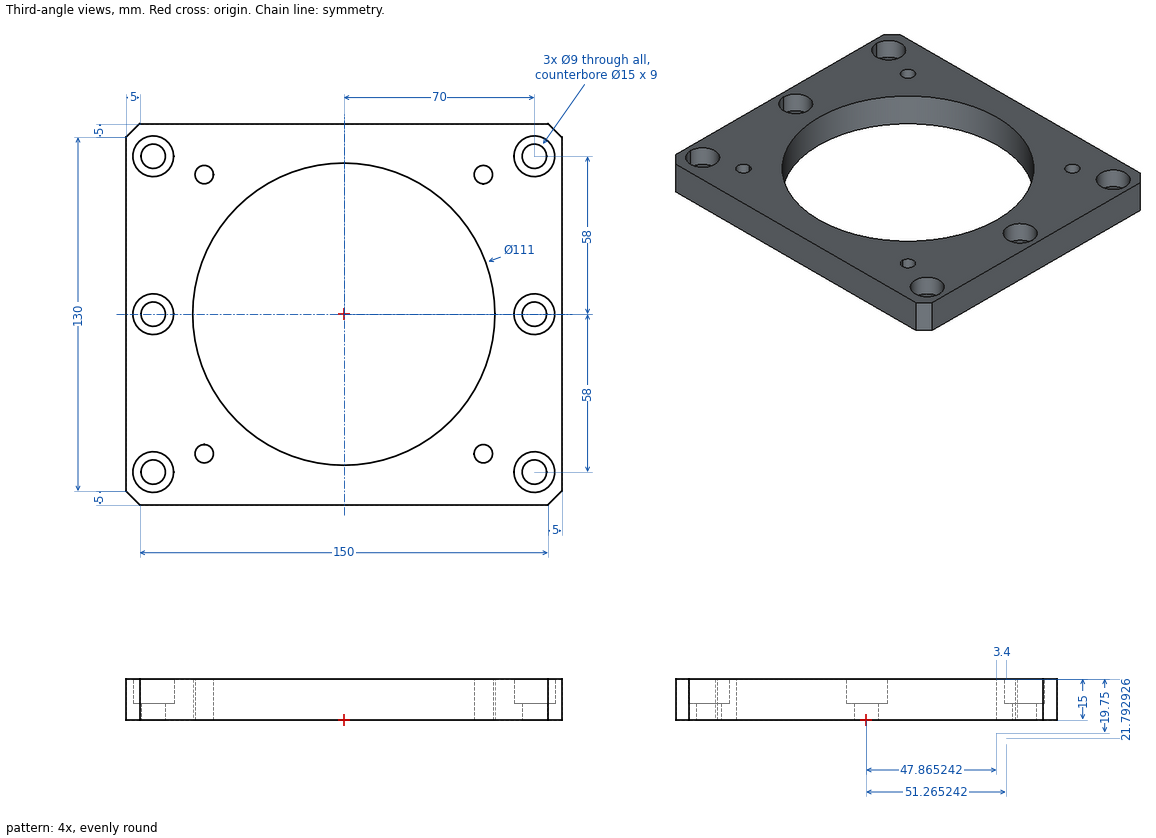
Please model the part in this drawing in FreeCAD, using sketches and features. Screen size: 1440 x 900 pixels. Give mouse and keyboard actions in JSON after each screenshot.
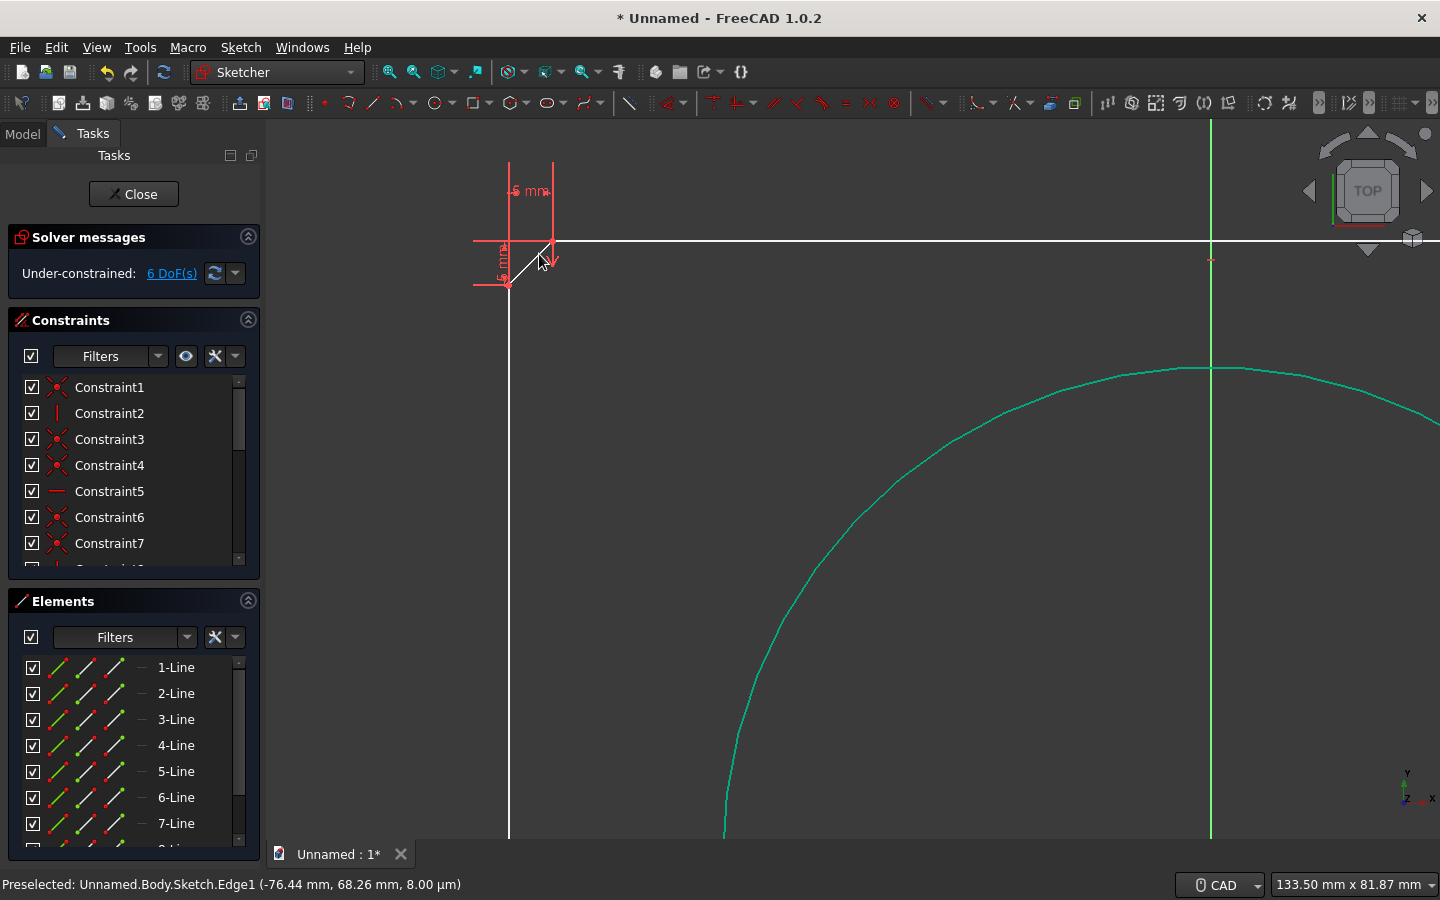
{"action": "scroll", "coordinate": [536, 260], "scroll_direction": "down", "scroll_amount": 5}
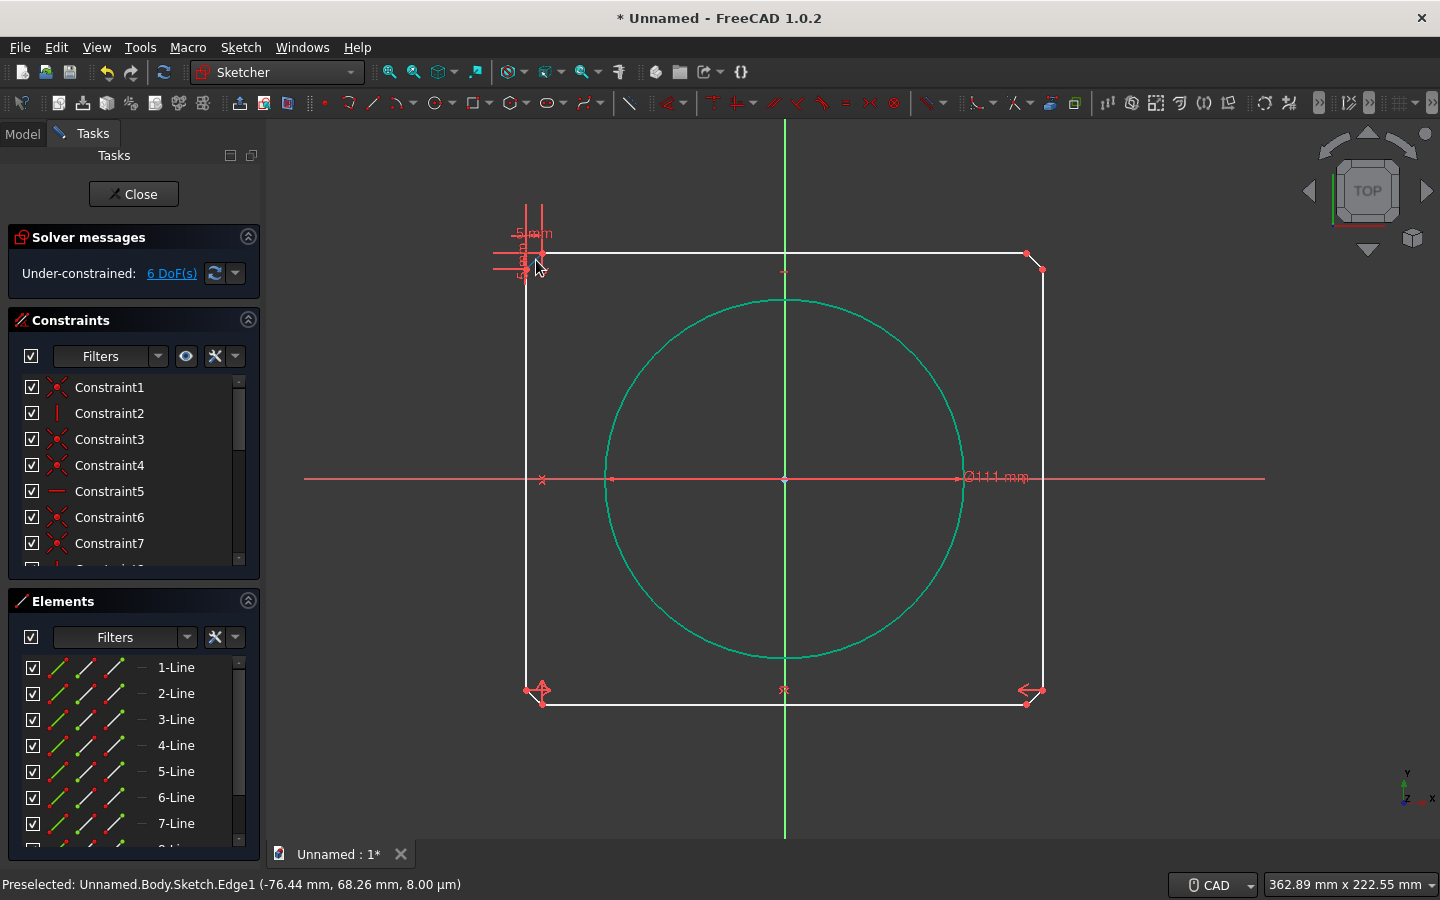
{"action": "scroll", "coordinate": [531, 695], "scroll_direction": "up", "scroll_amount": 5}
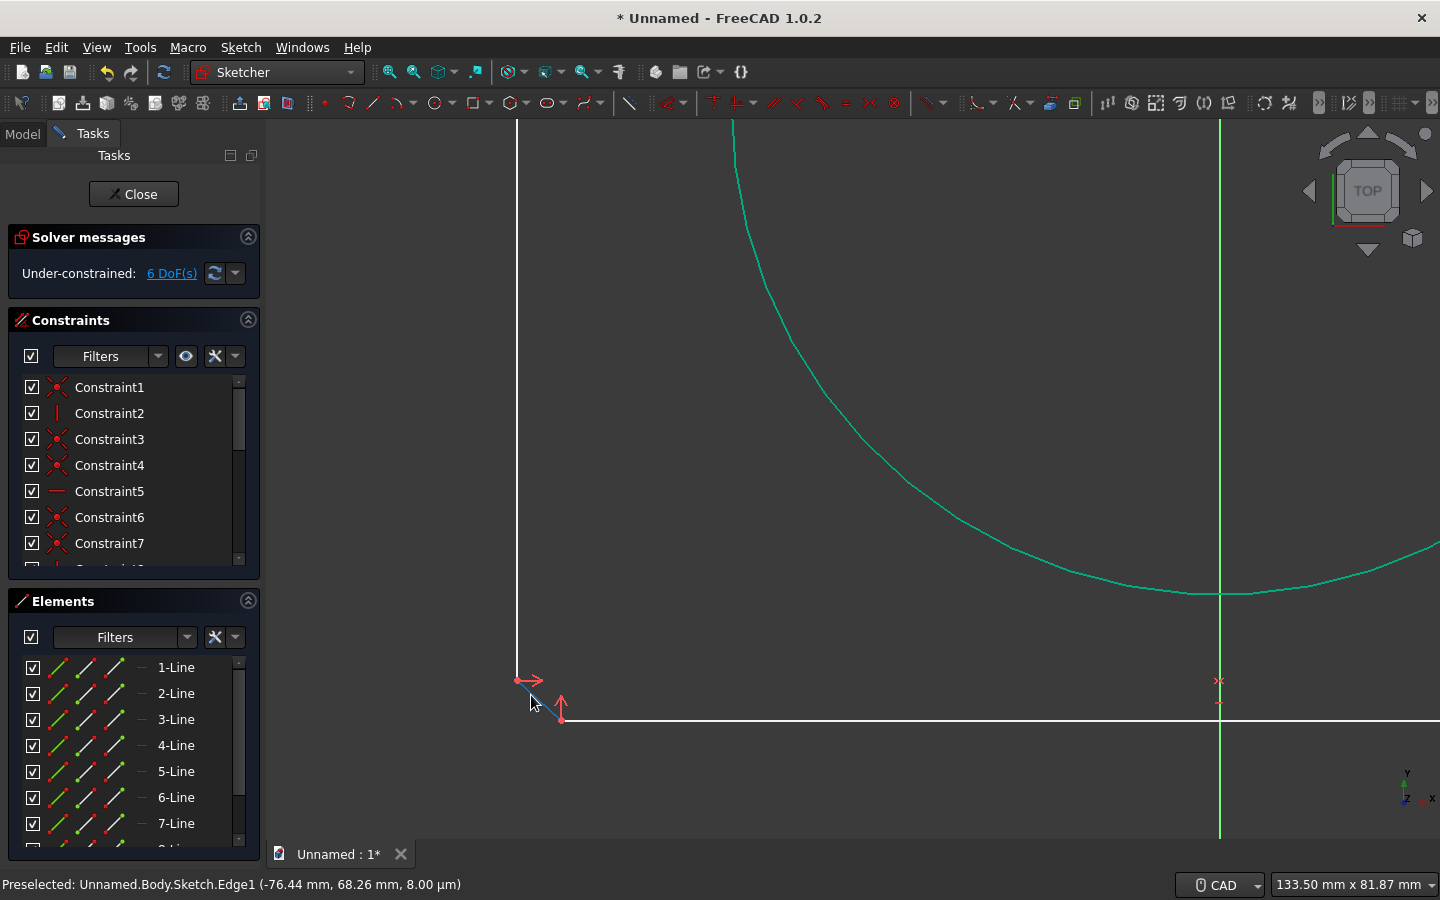
{"action": "left_click", "coordinate": [530, 693]}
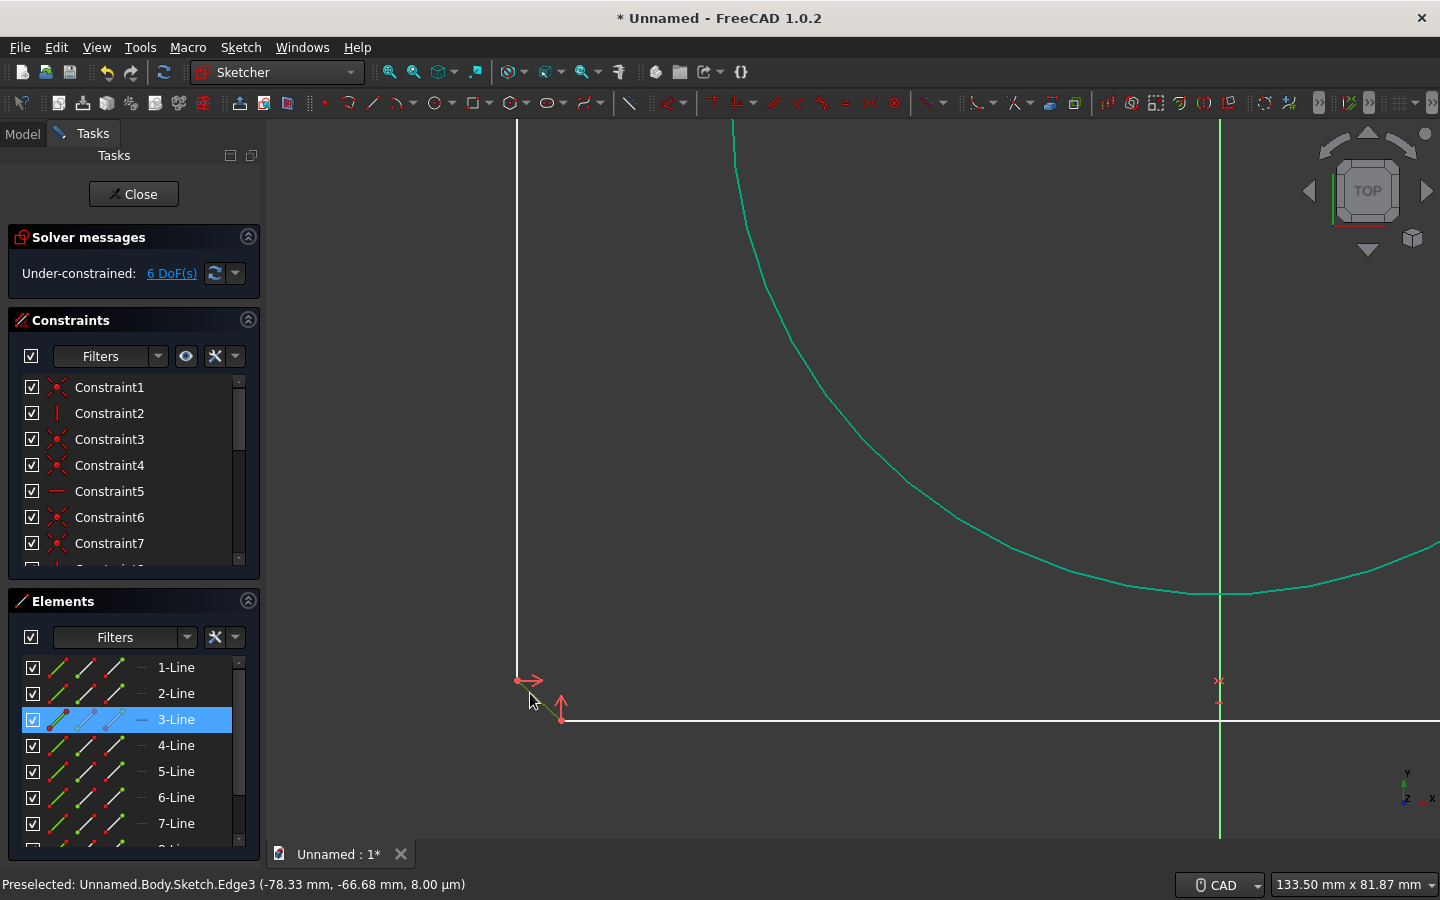
{"action": "left_click", "coordinate": [686, 104]}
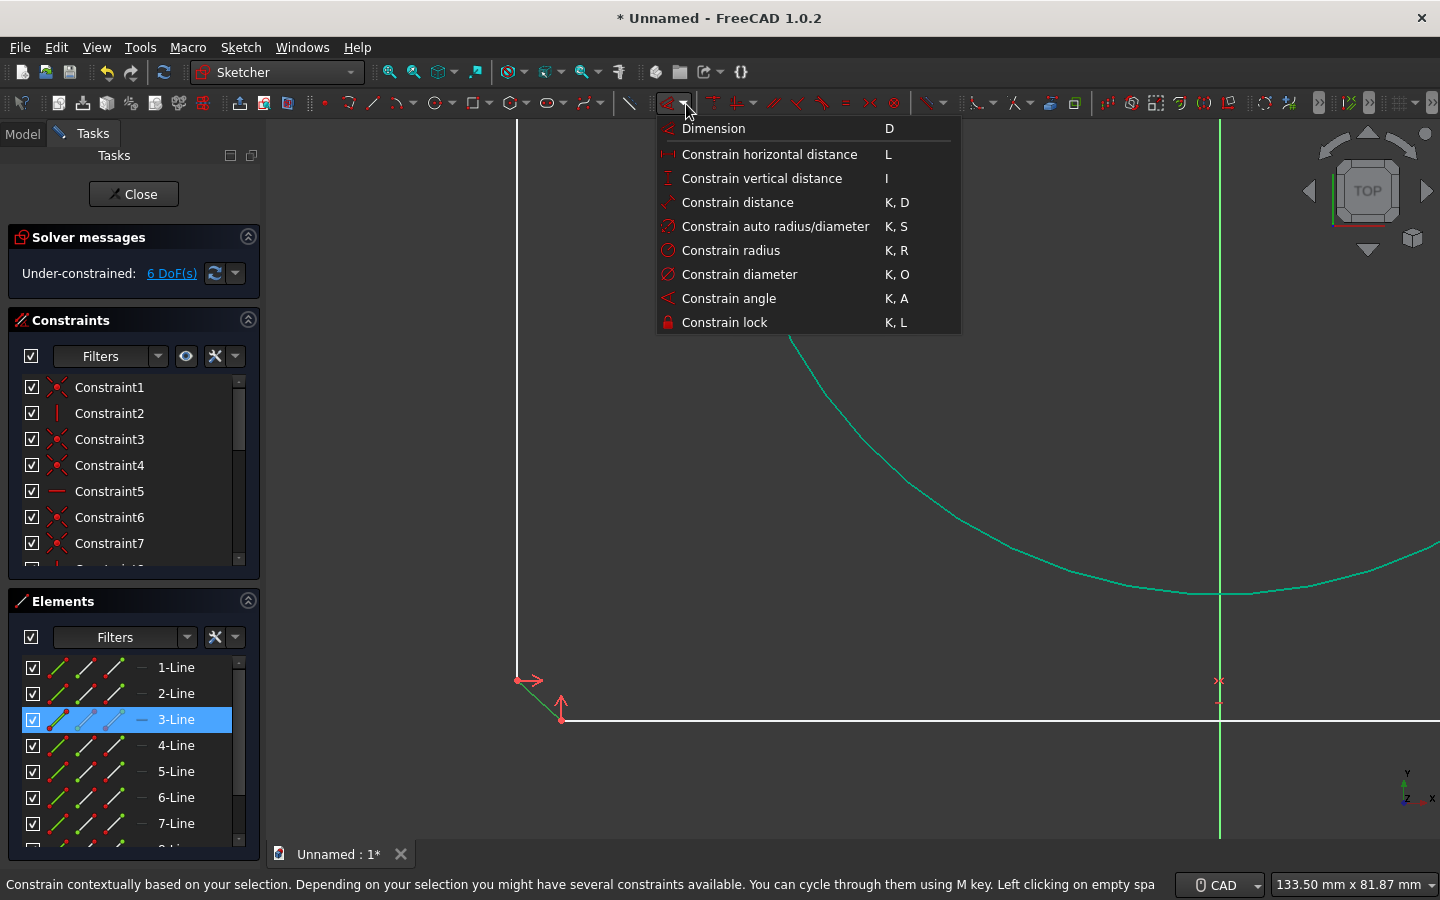
{"action": "left_click", "coordinate": [809, 178]}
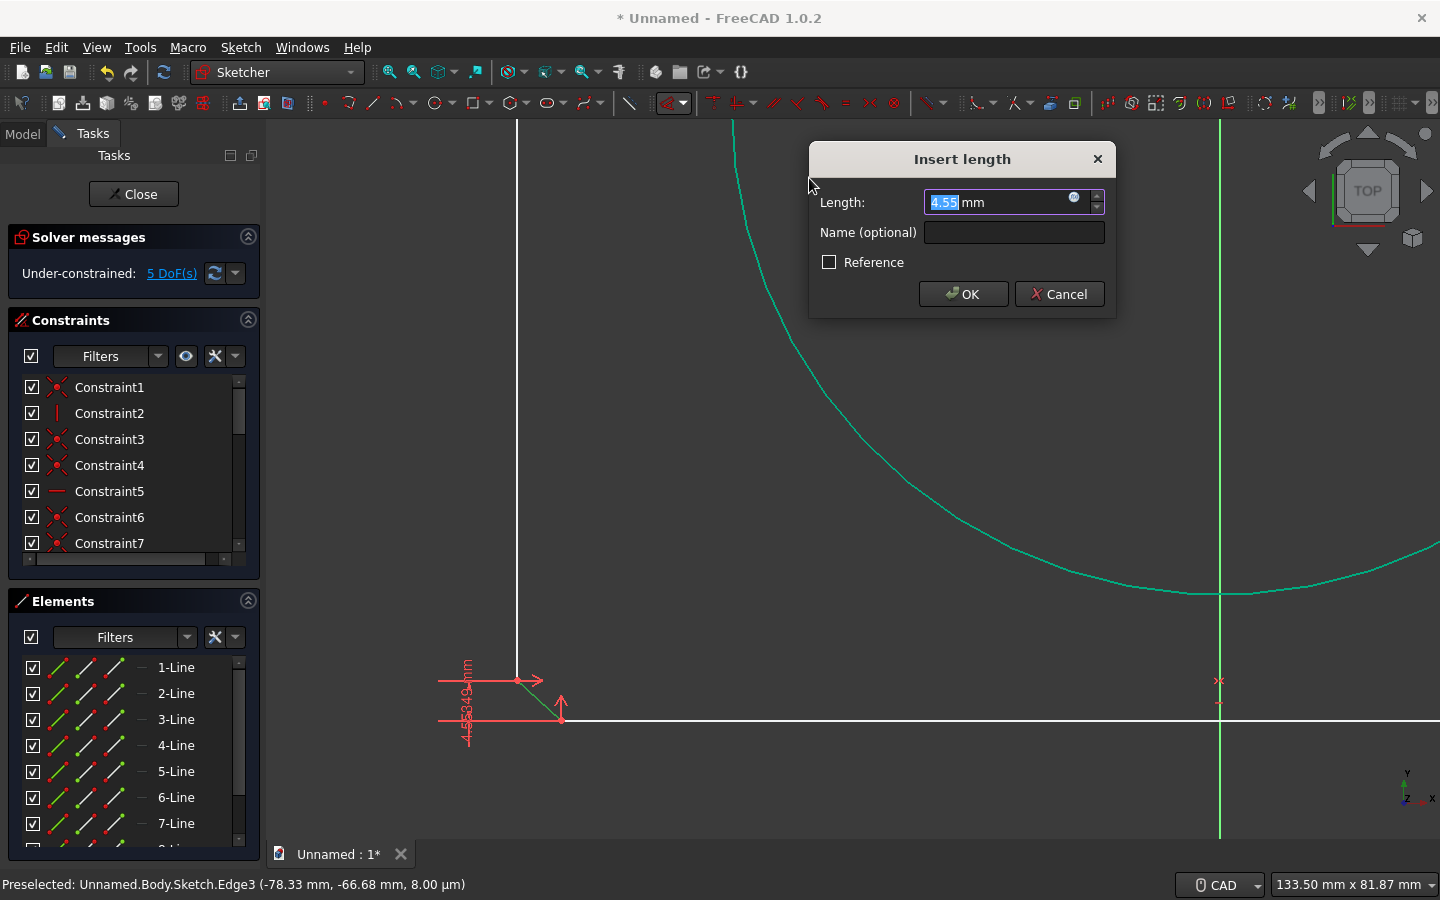
{"action": "type", "text": "5"}
{"action": "key", "text": "Return"}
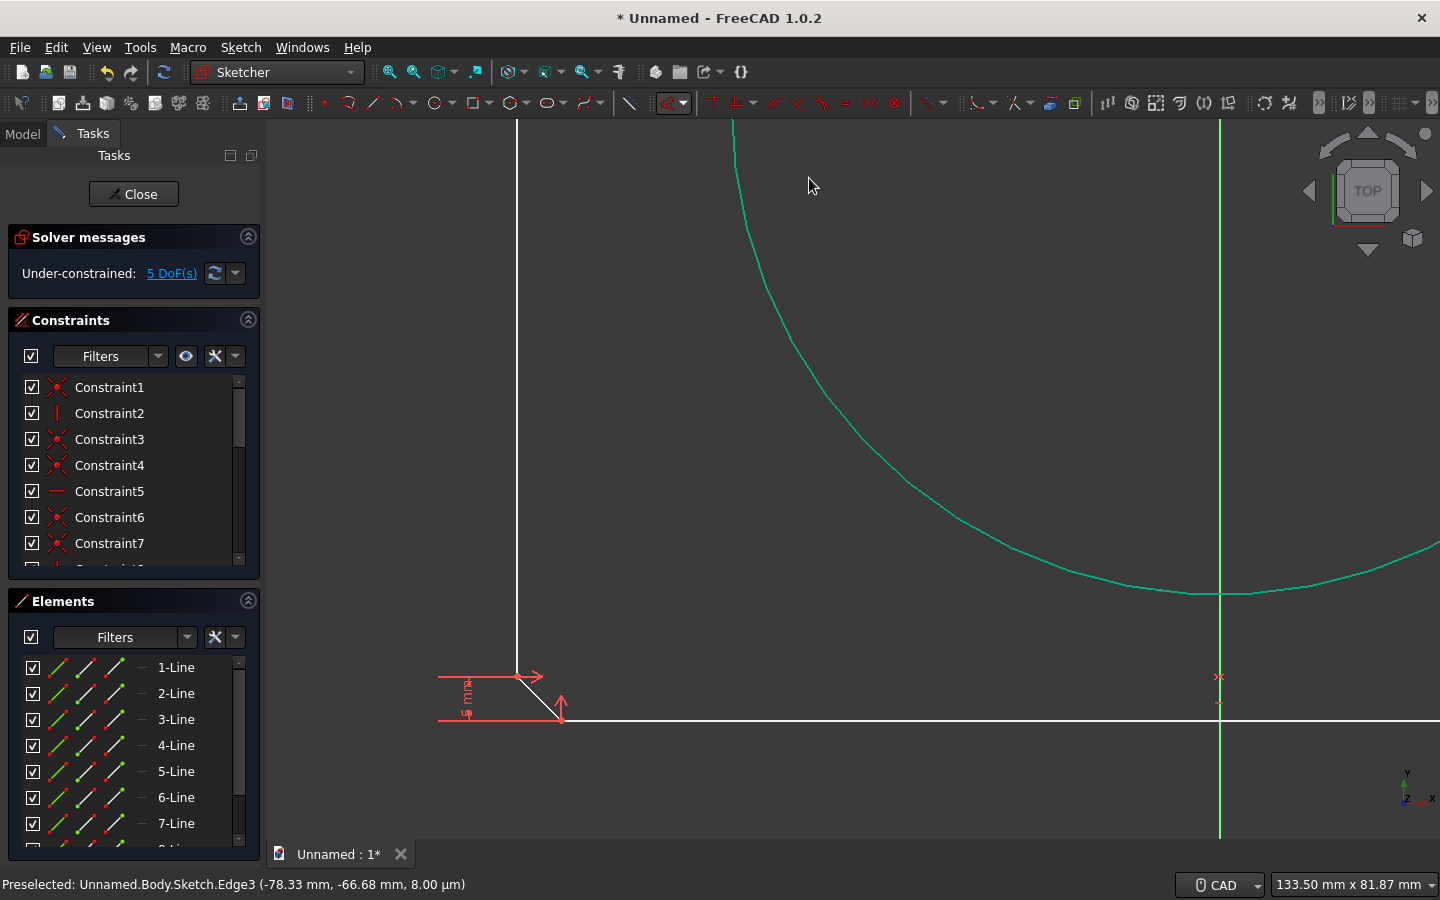
{"action": "scroll", "coordinate": [531, 696], "scroll_direction": "down", "scroll_amount": 5}